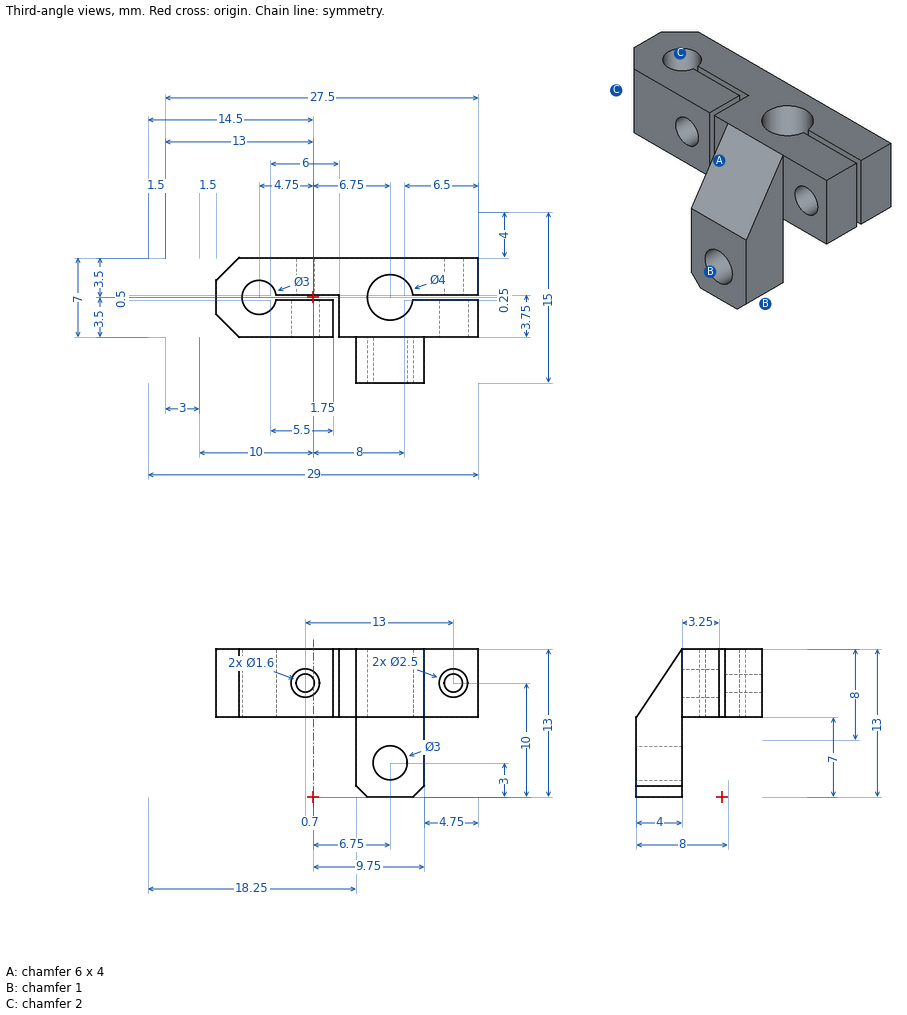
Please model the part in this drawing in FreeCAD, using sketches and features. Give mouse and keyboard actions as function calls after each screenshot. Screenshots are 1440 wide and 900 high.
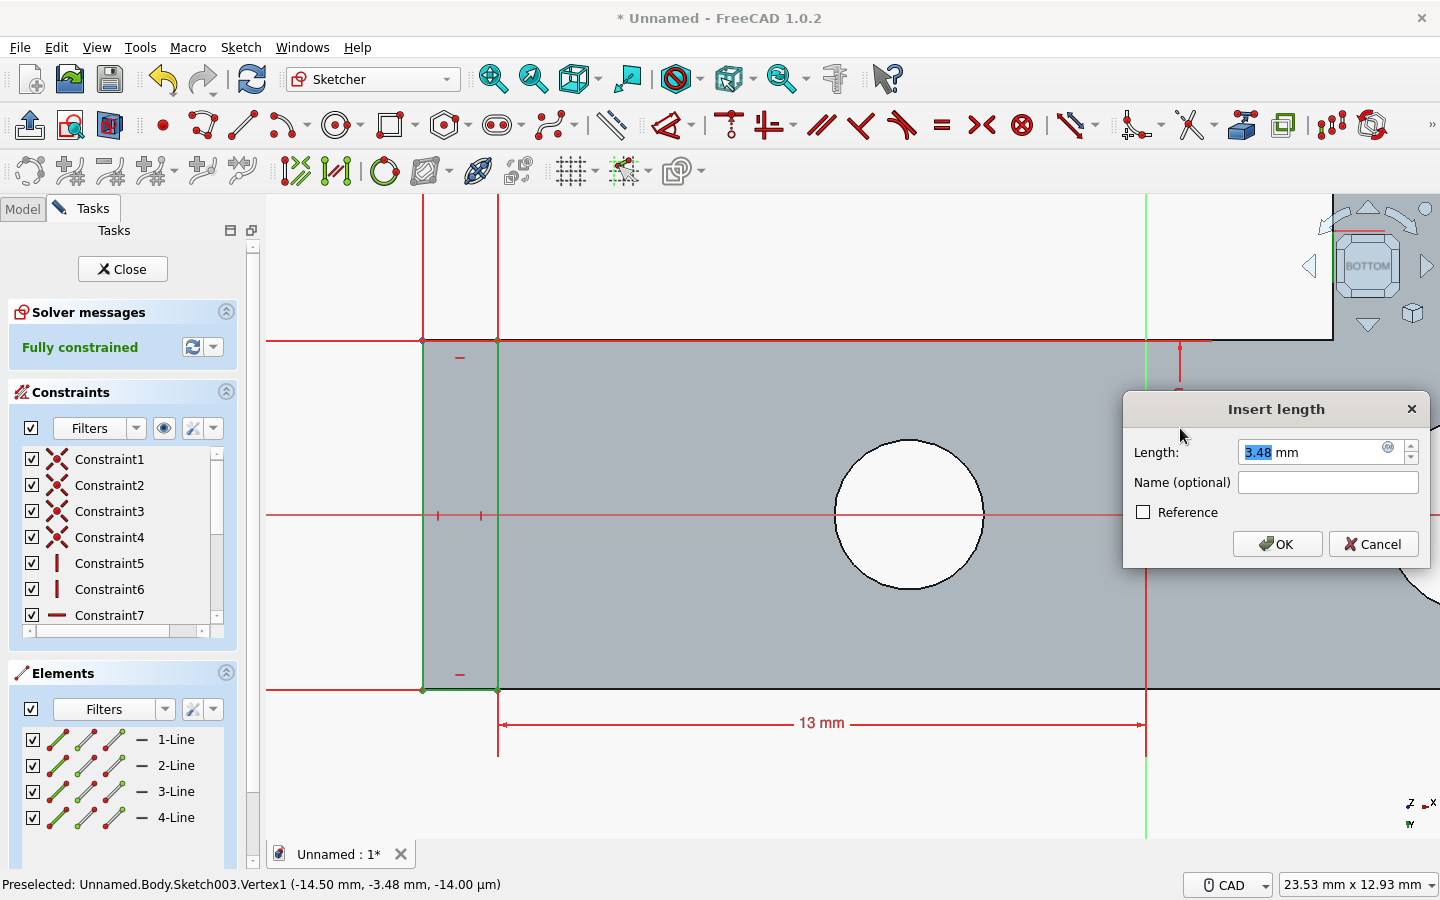
text(3.5)
key(Return)
key(Escape)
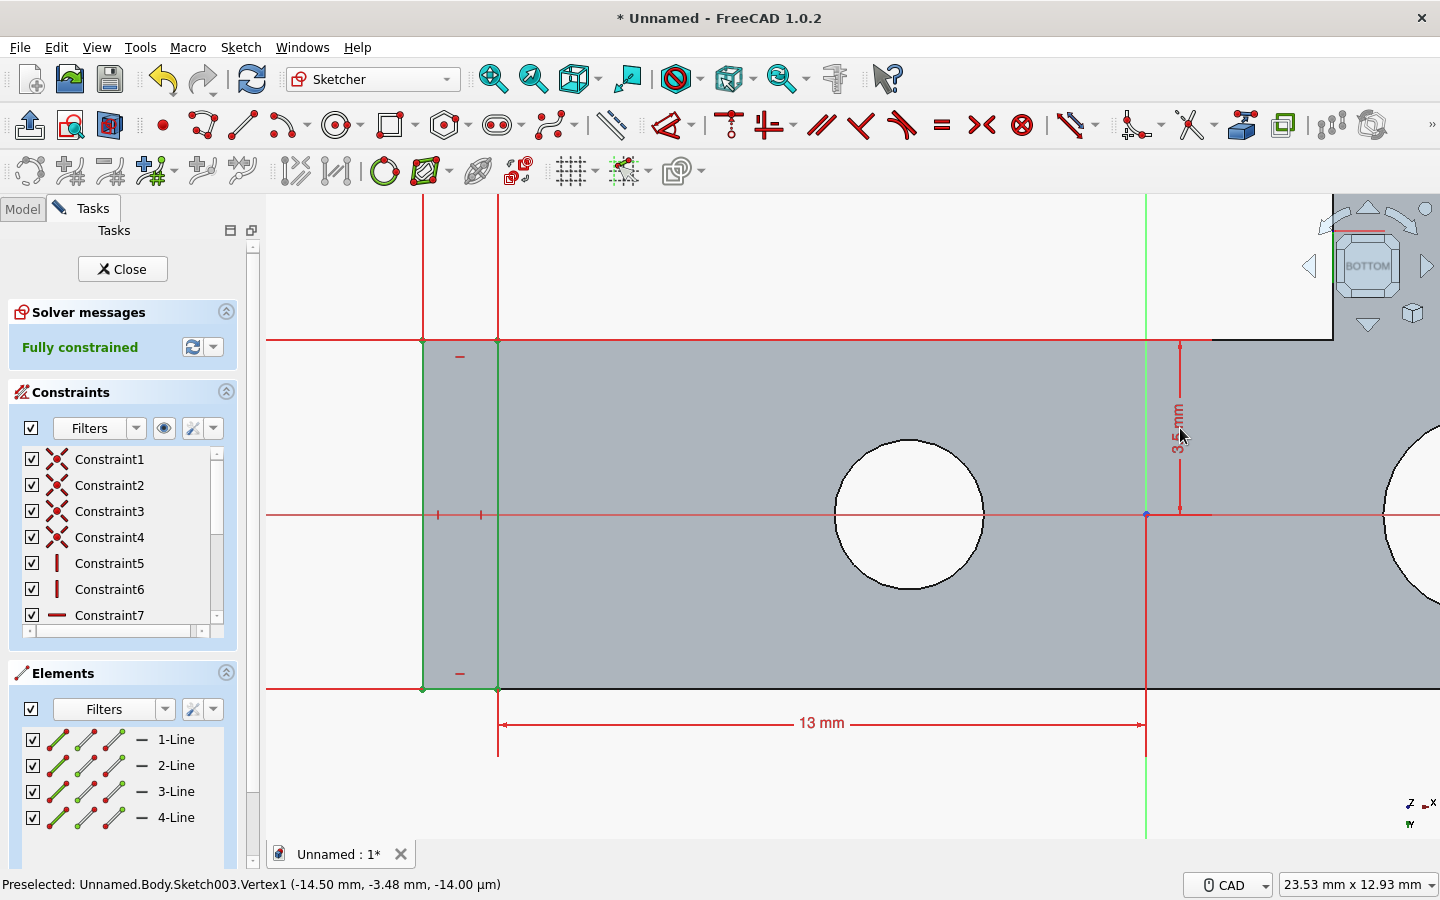
click(123, 269)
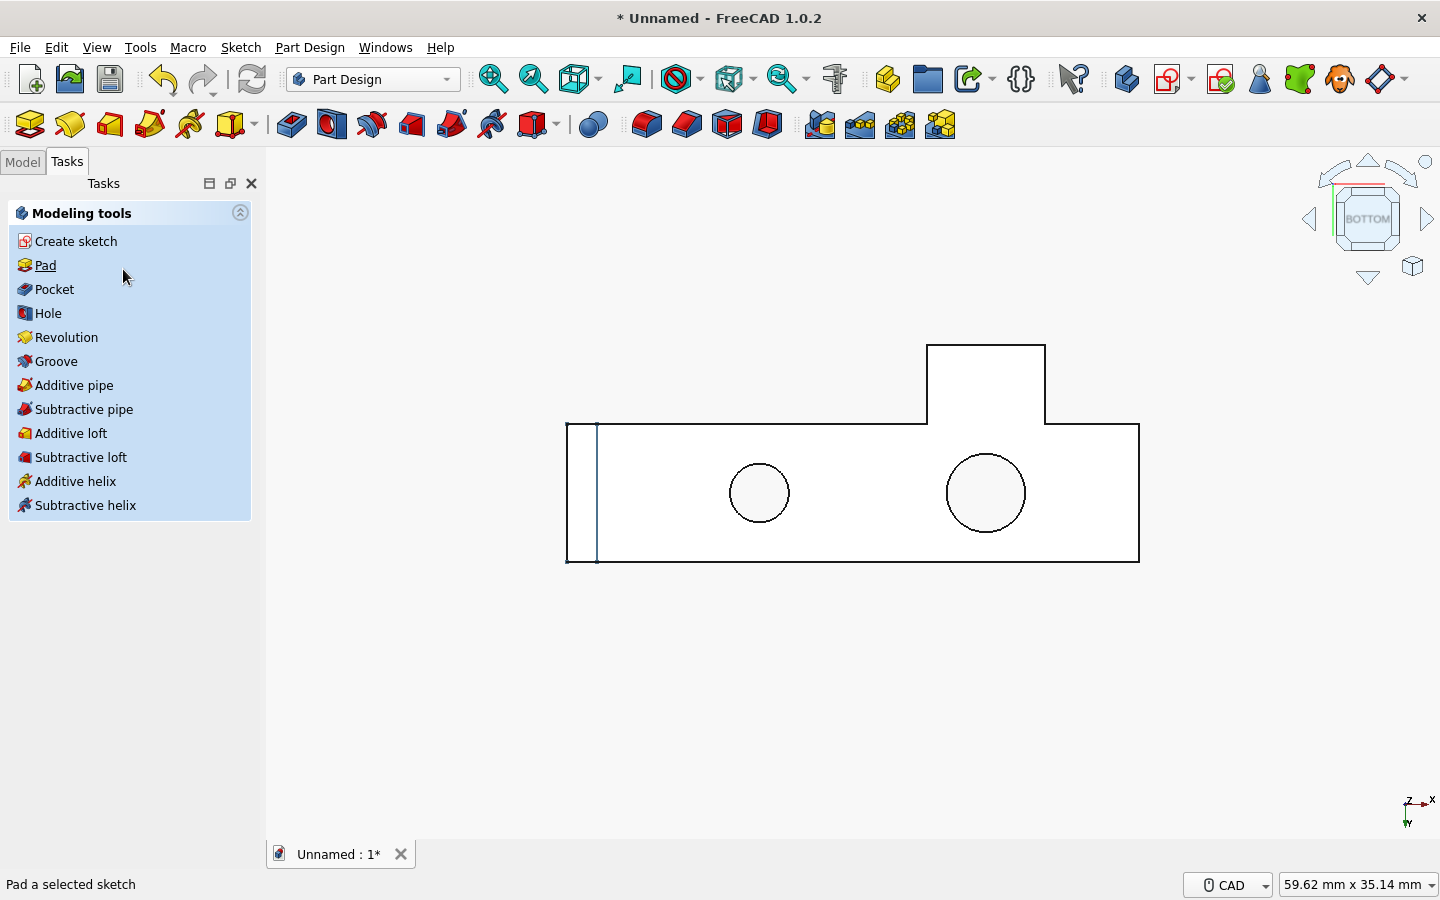
click(292, 124)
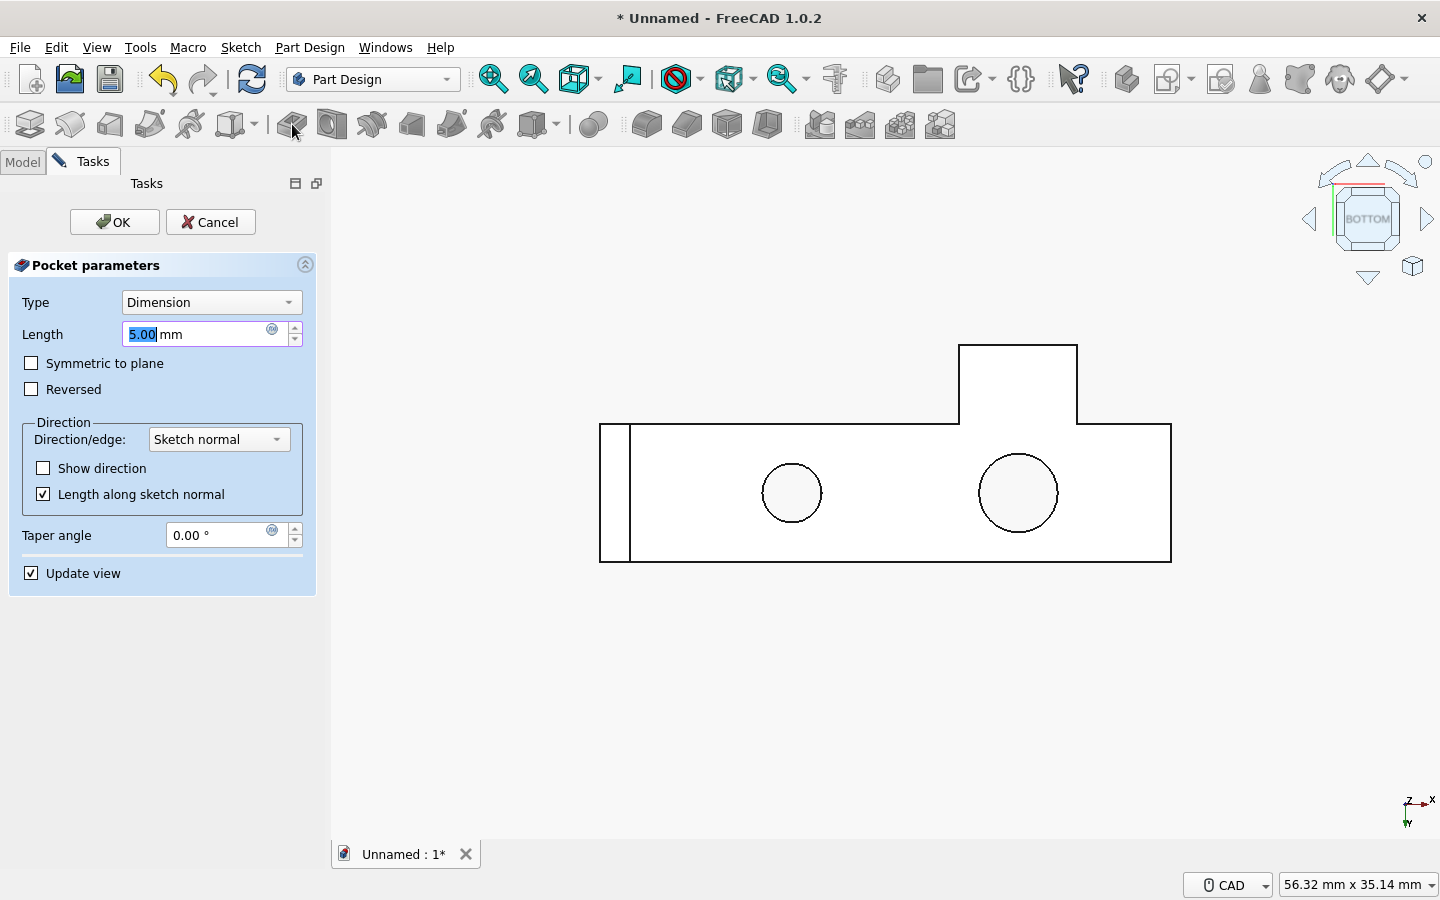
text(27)
key(Tab)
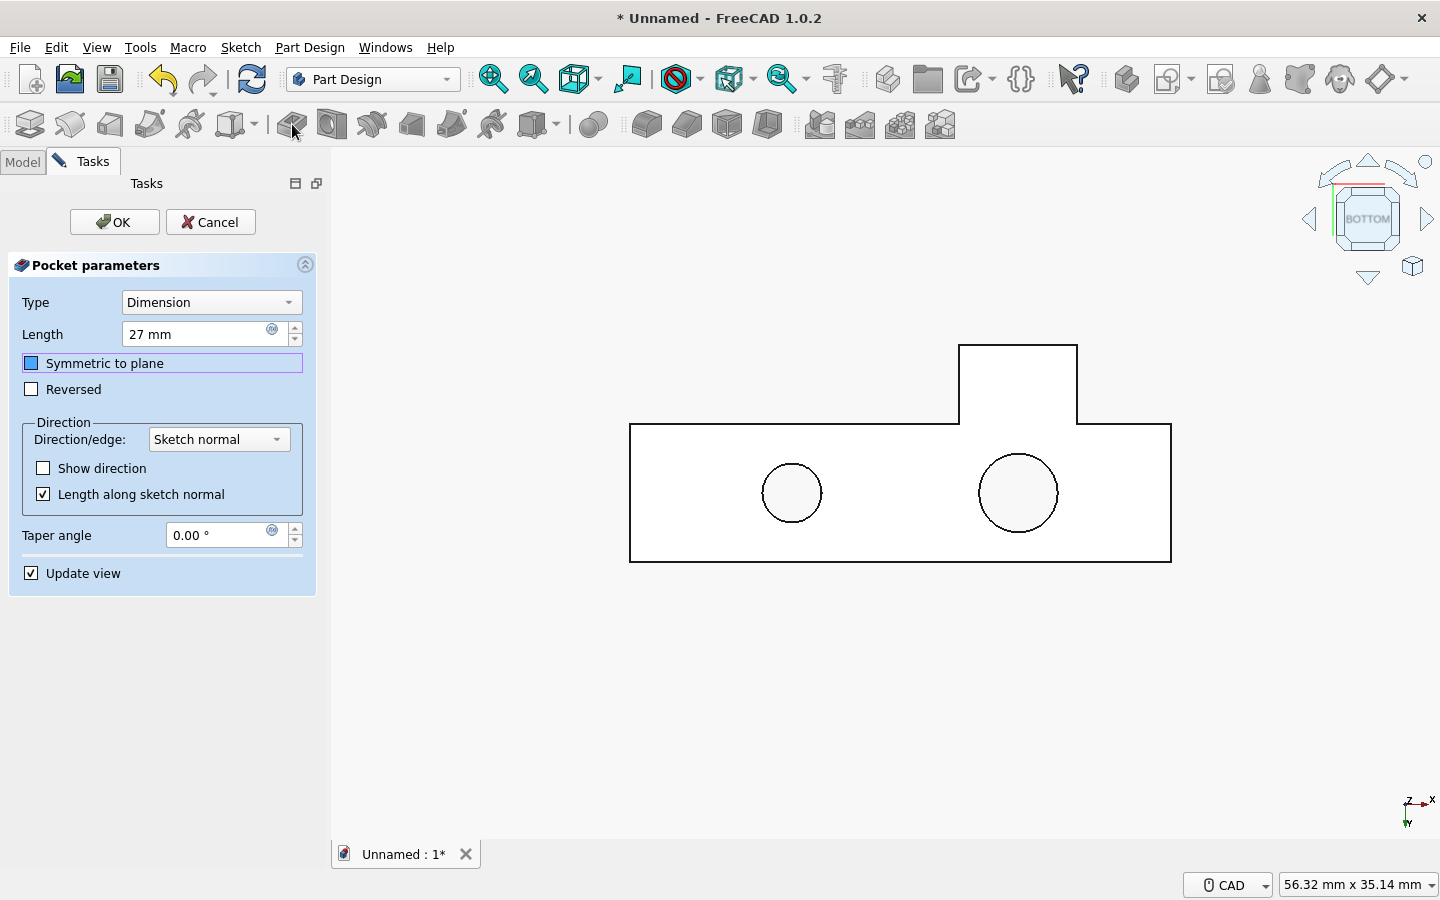
click(115, 222)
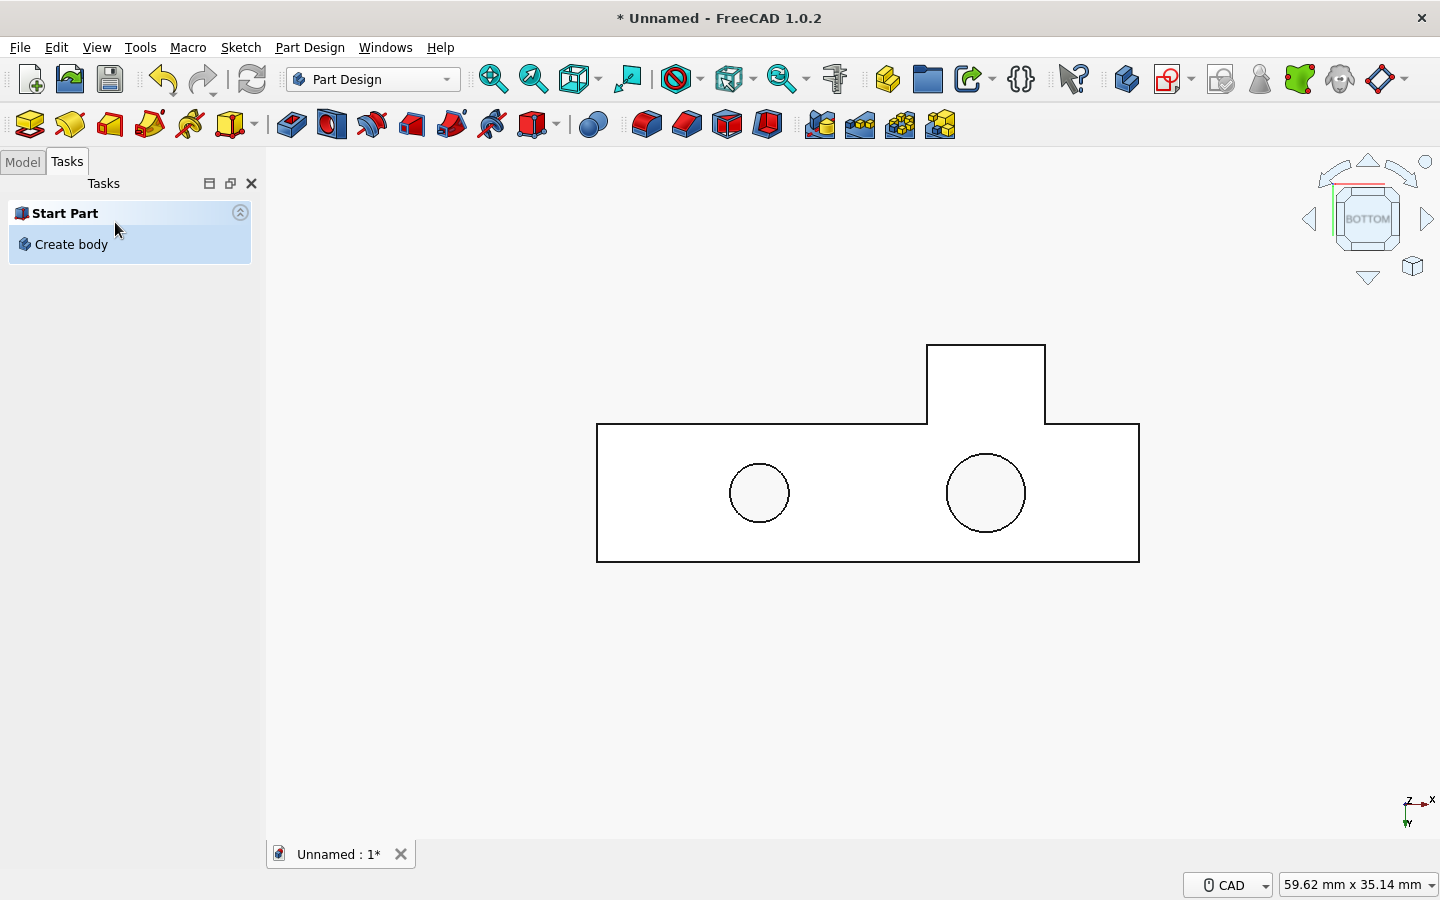
click(868, 484)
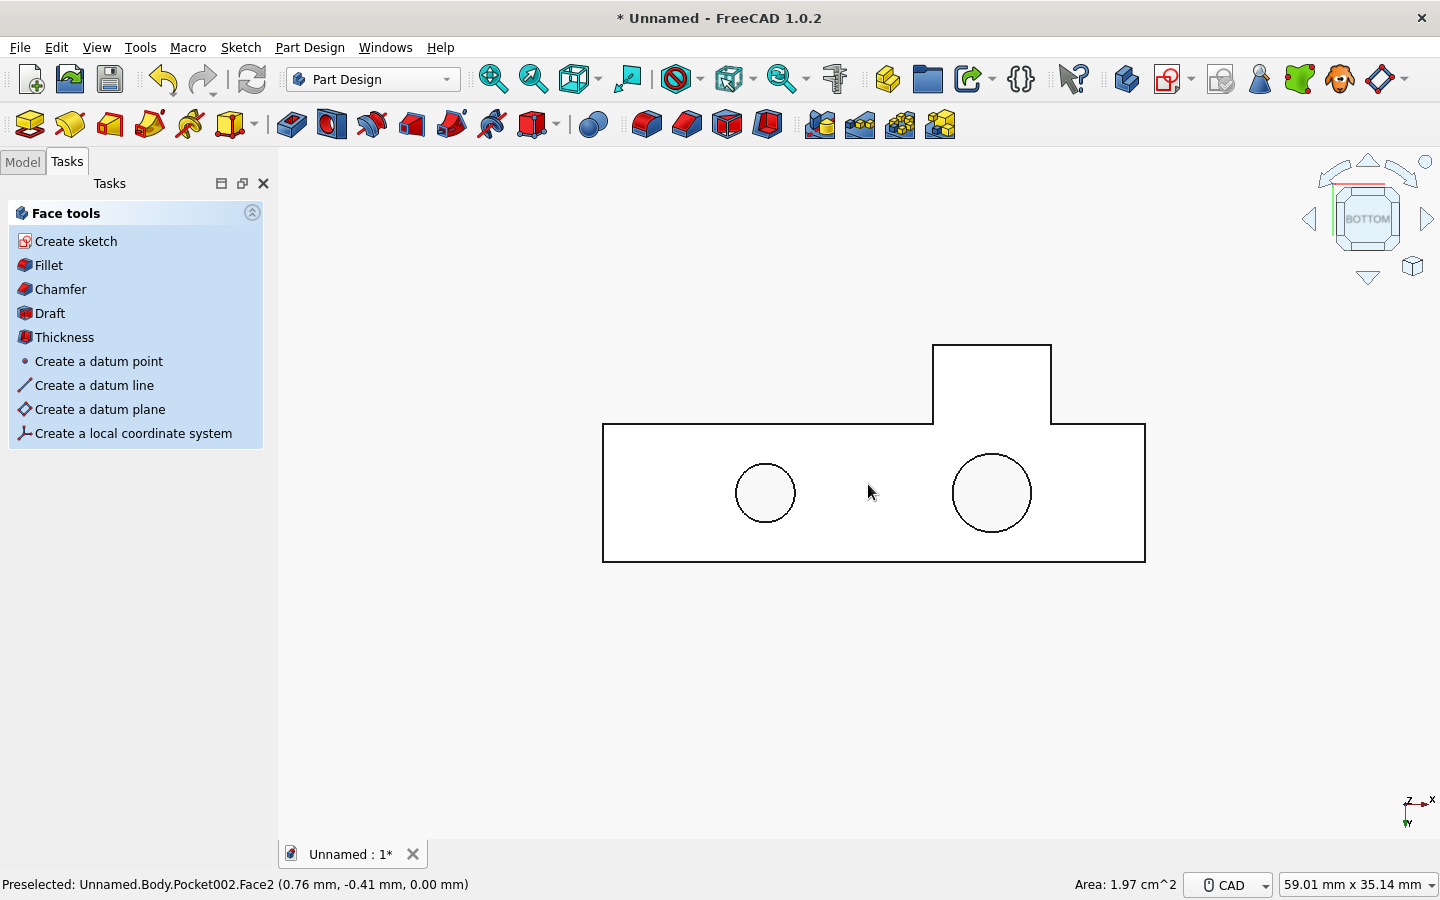
click(1168, 80)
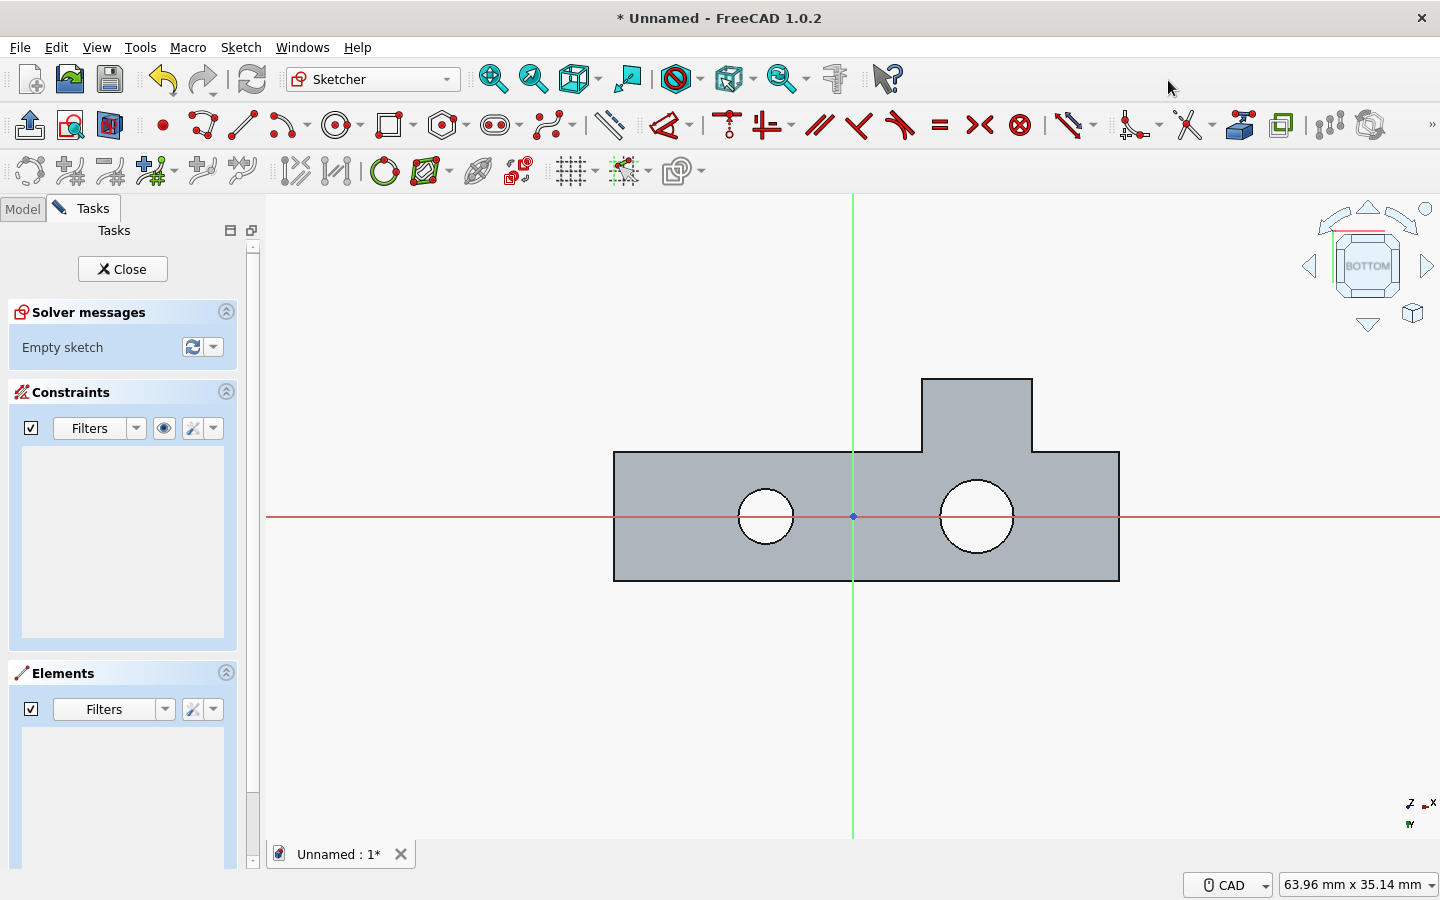
scroll(1034, 517, up, 2)